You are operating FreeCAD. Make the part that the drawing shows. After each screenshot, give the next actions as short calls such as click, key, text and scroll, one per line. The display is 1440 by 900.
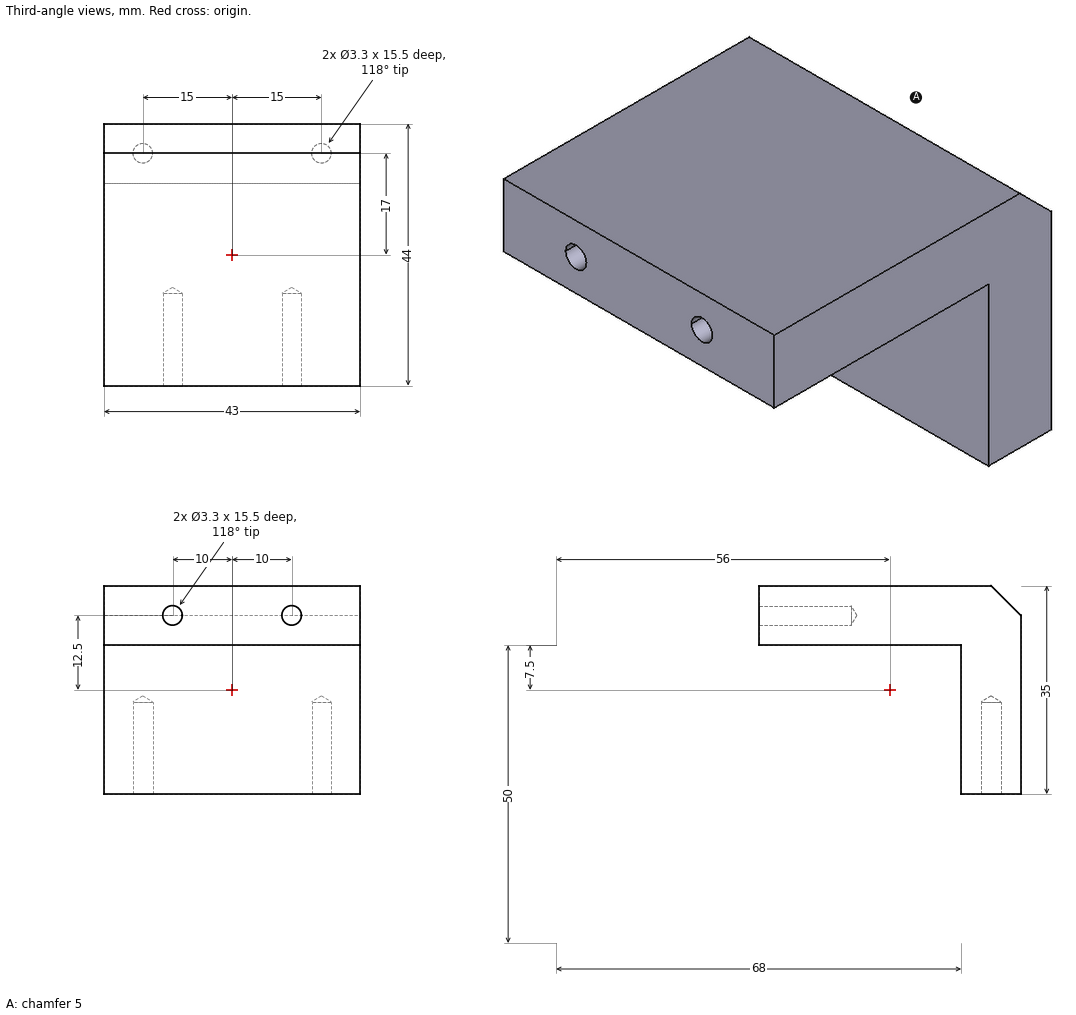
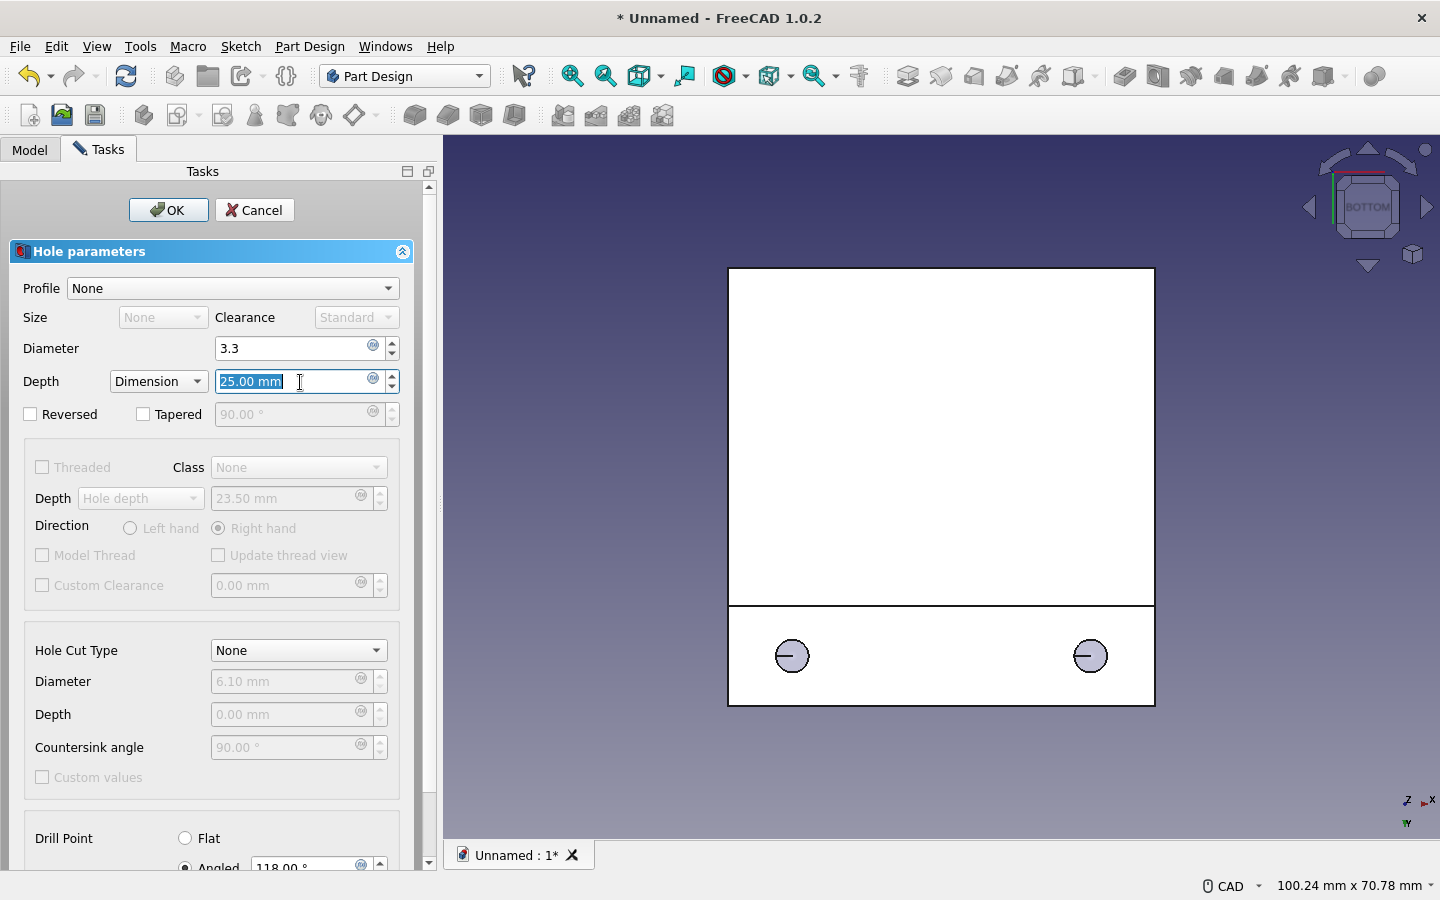
text(15.5)
key(Tab)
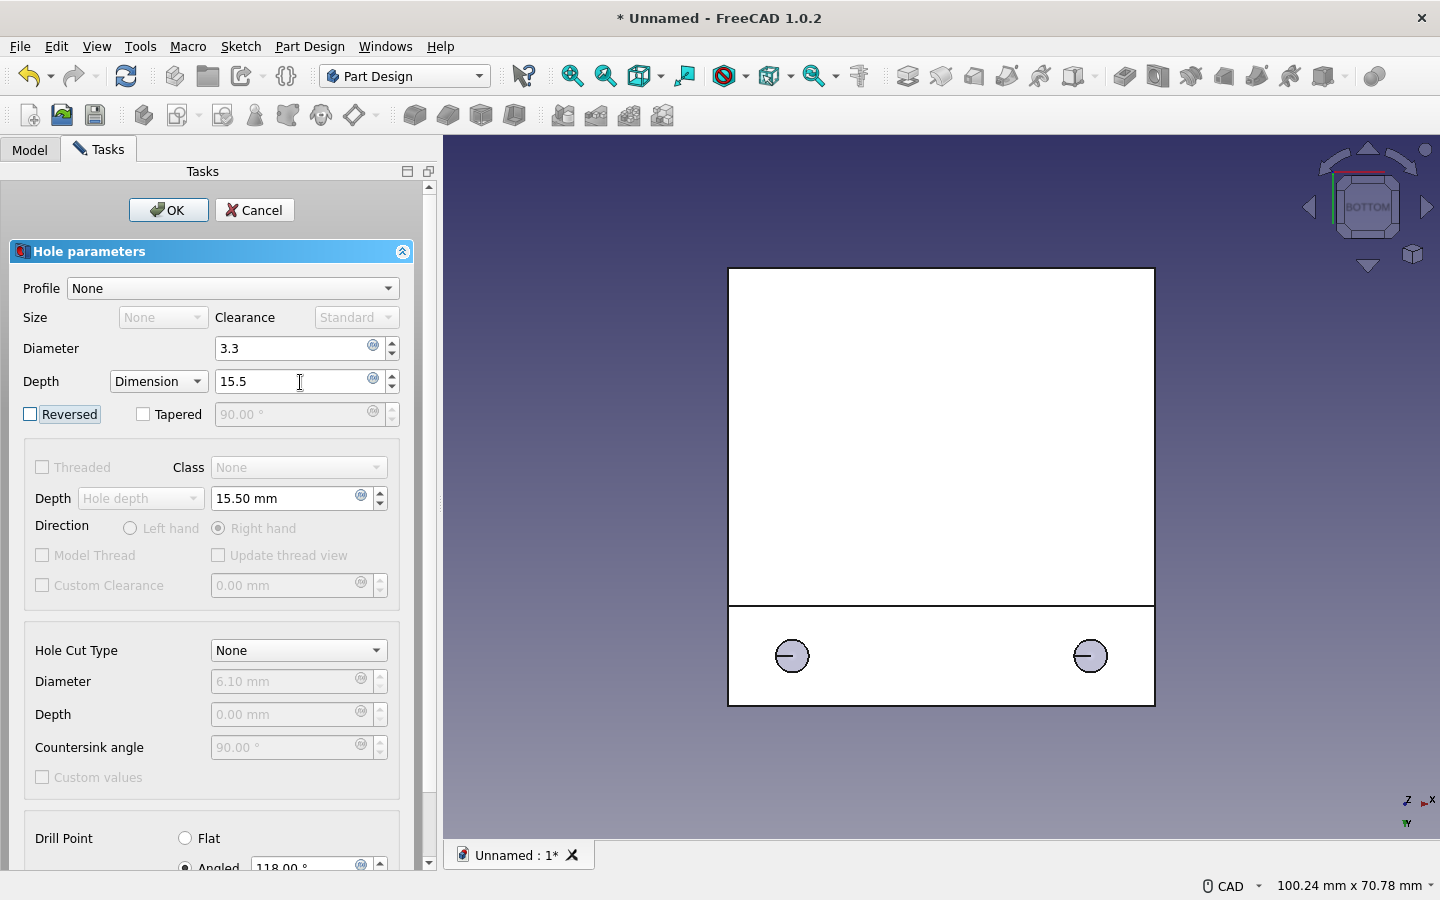
click(169, 210)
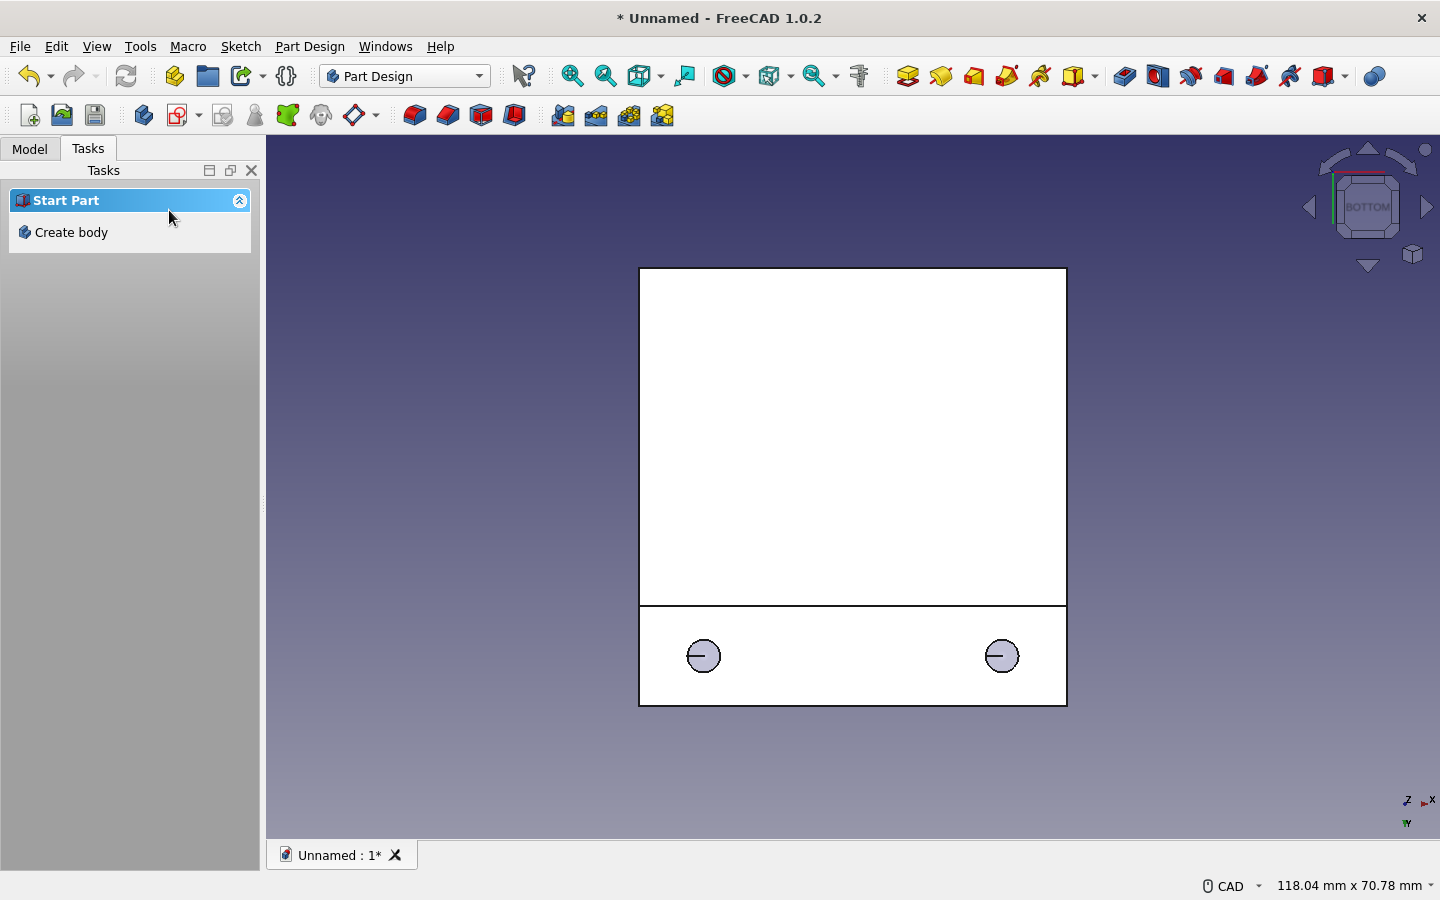
key(0)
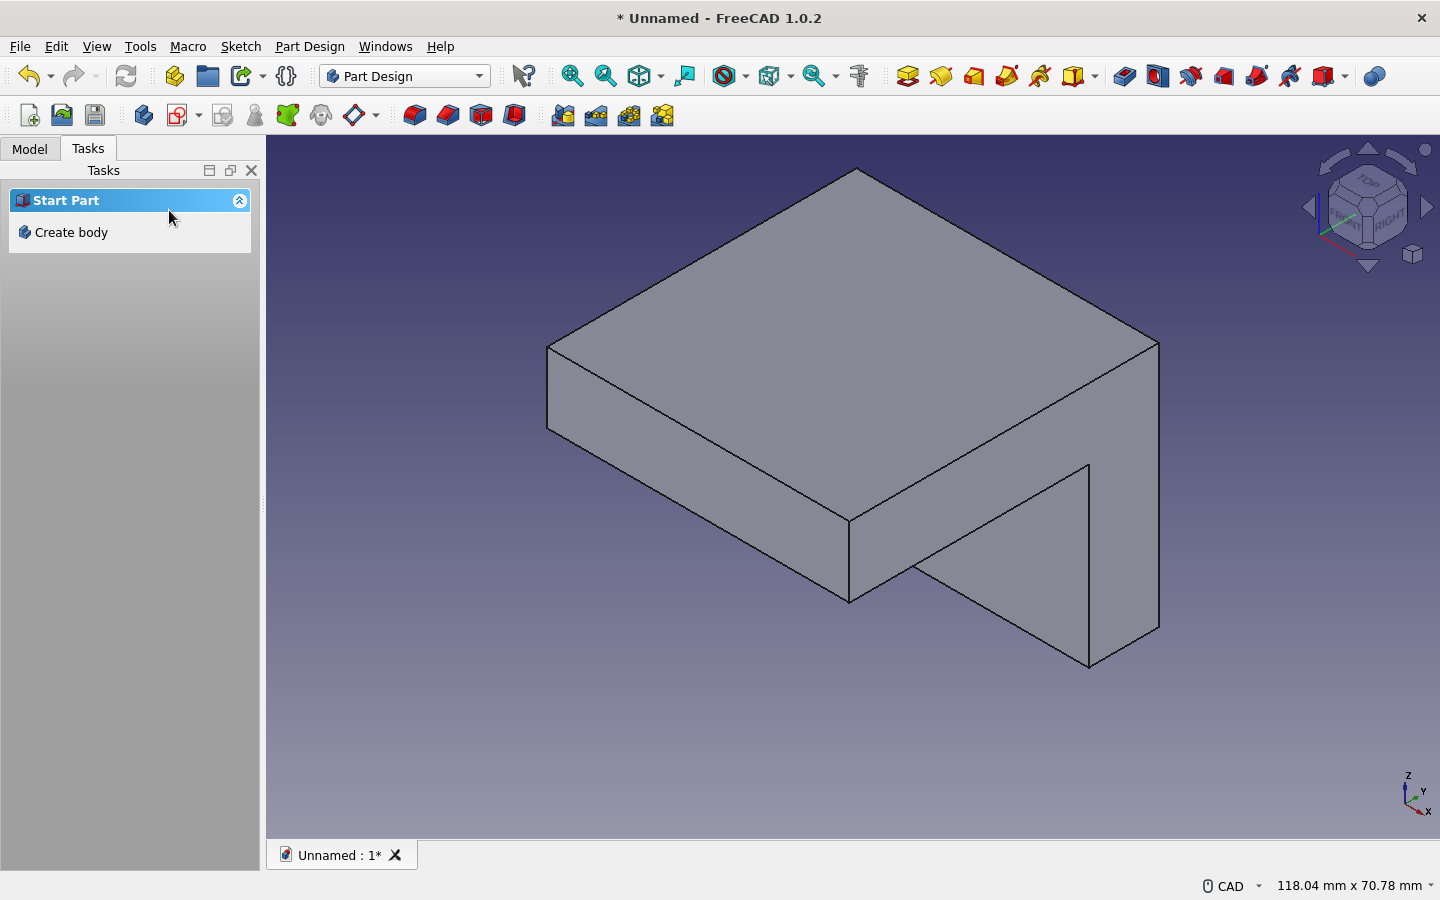
key(2)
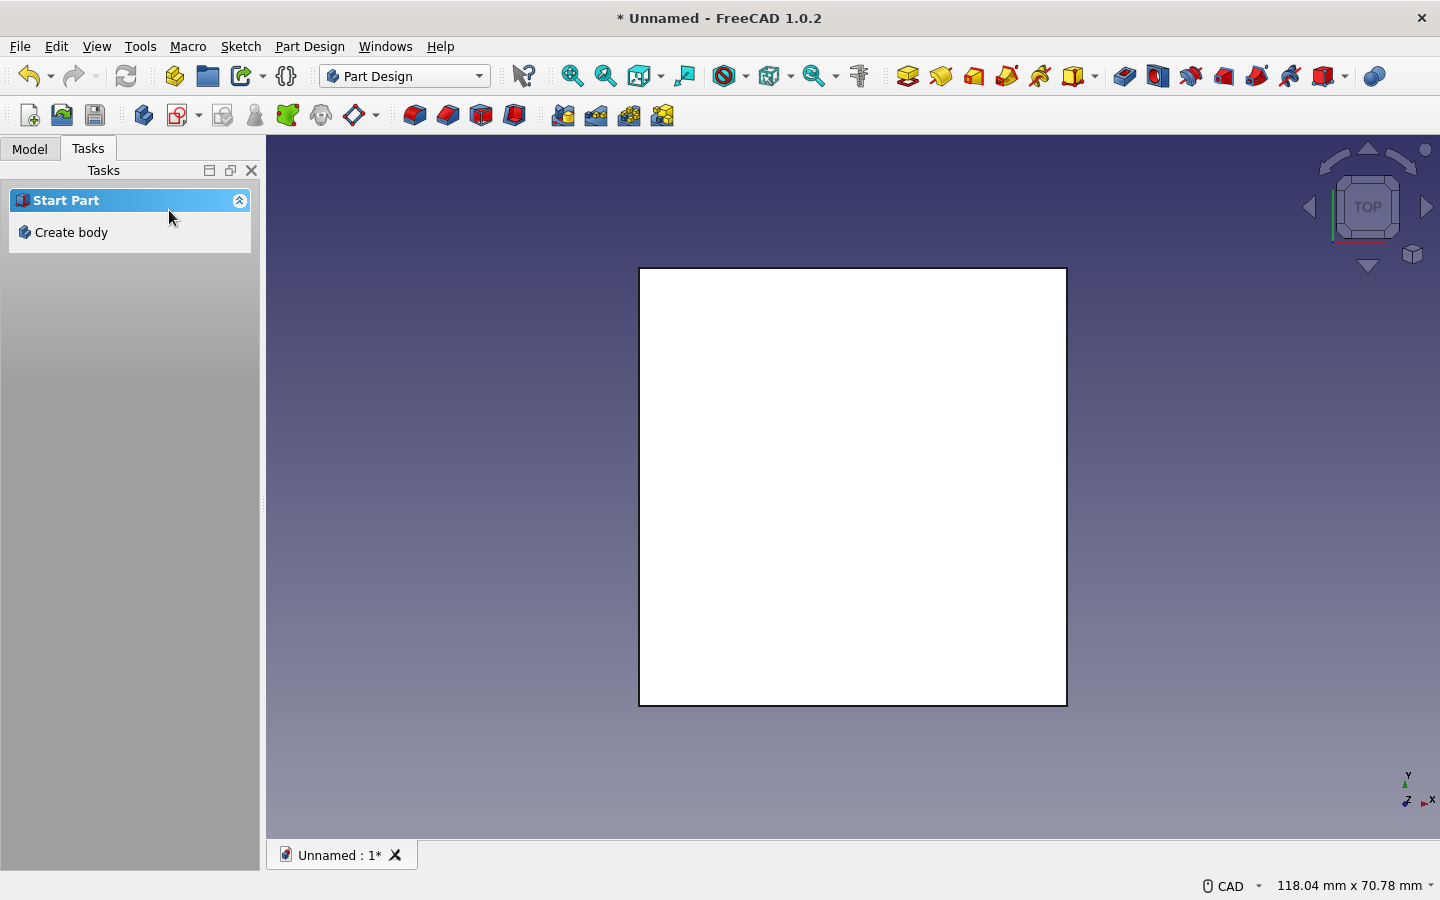
click(853, 267)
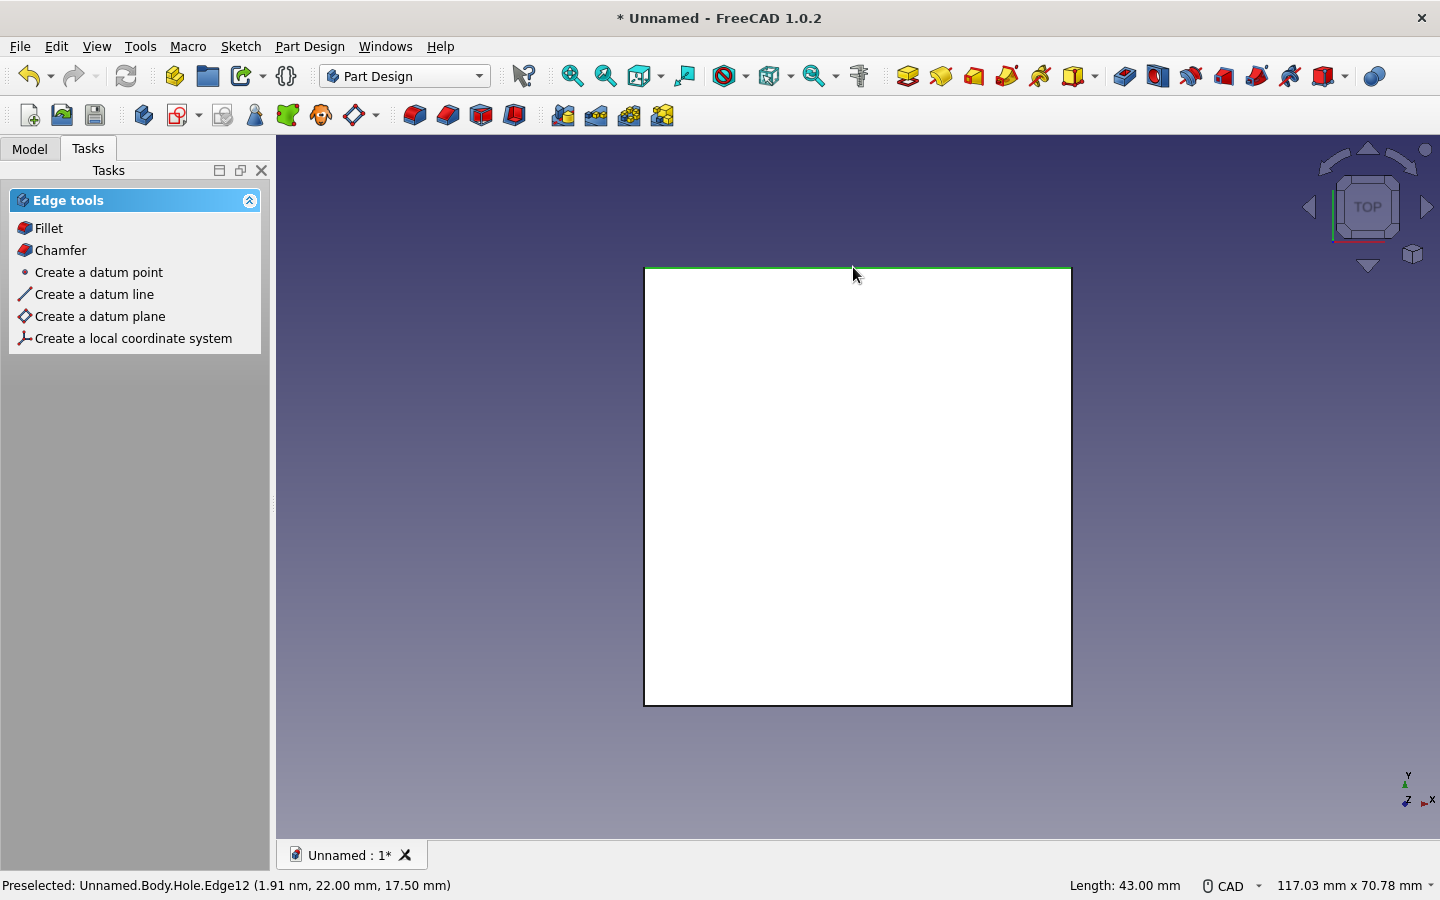
click(448, 116)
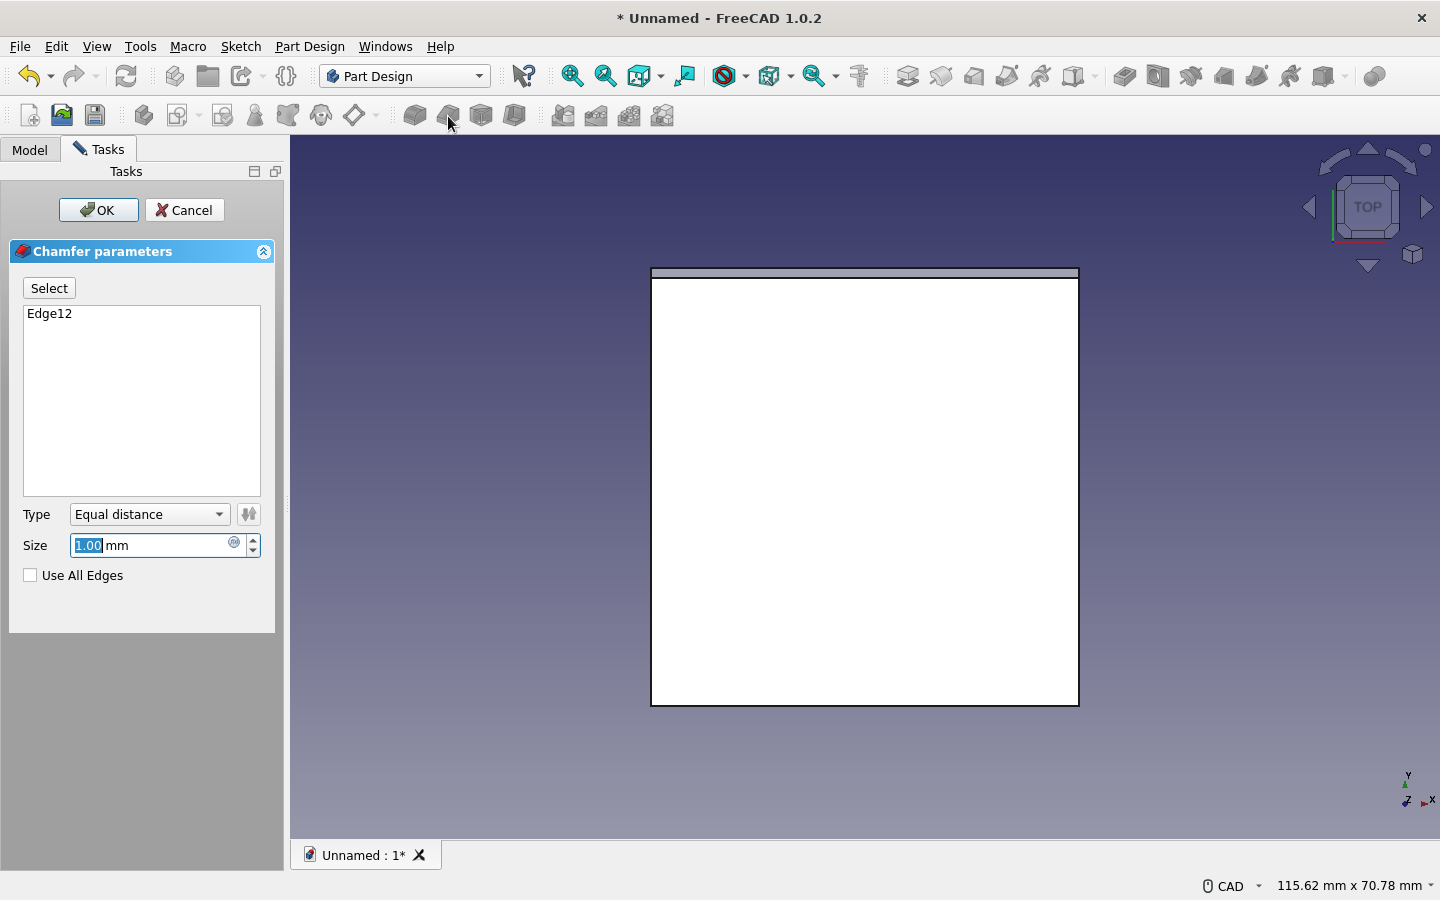
text(5)
key(Tab)